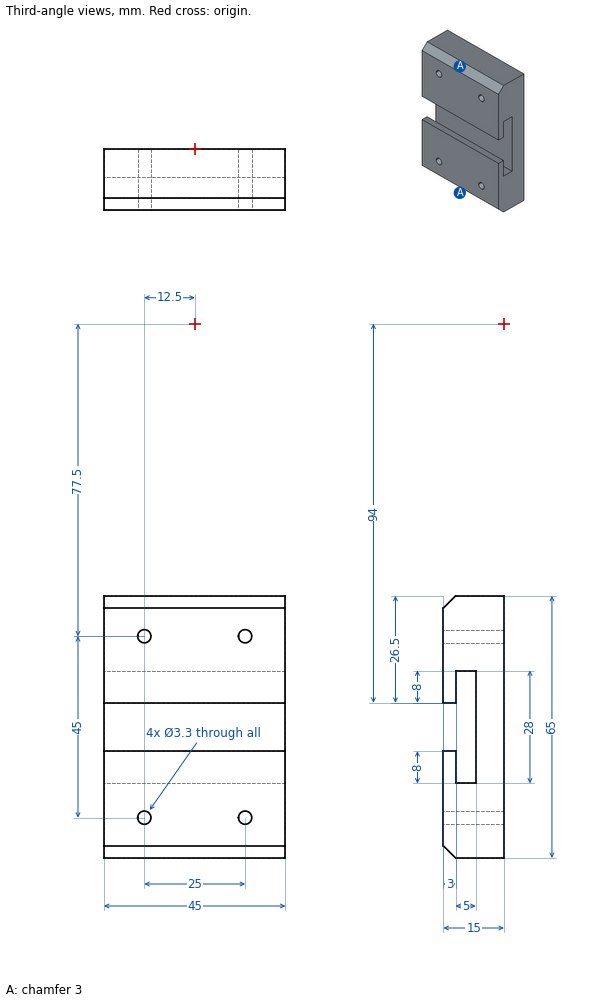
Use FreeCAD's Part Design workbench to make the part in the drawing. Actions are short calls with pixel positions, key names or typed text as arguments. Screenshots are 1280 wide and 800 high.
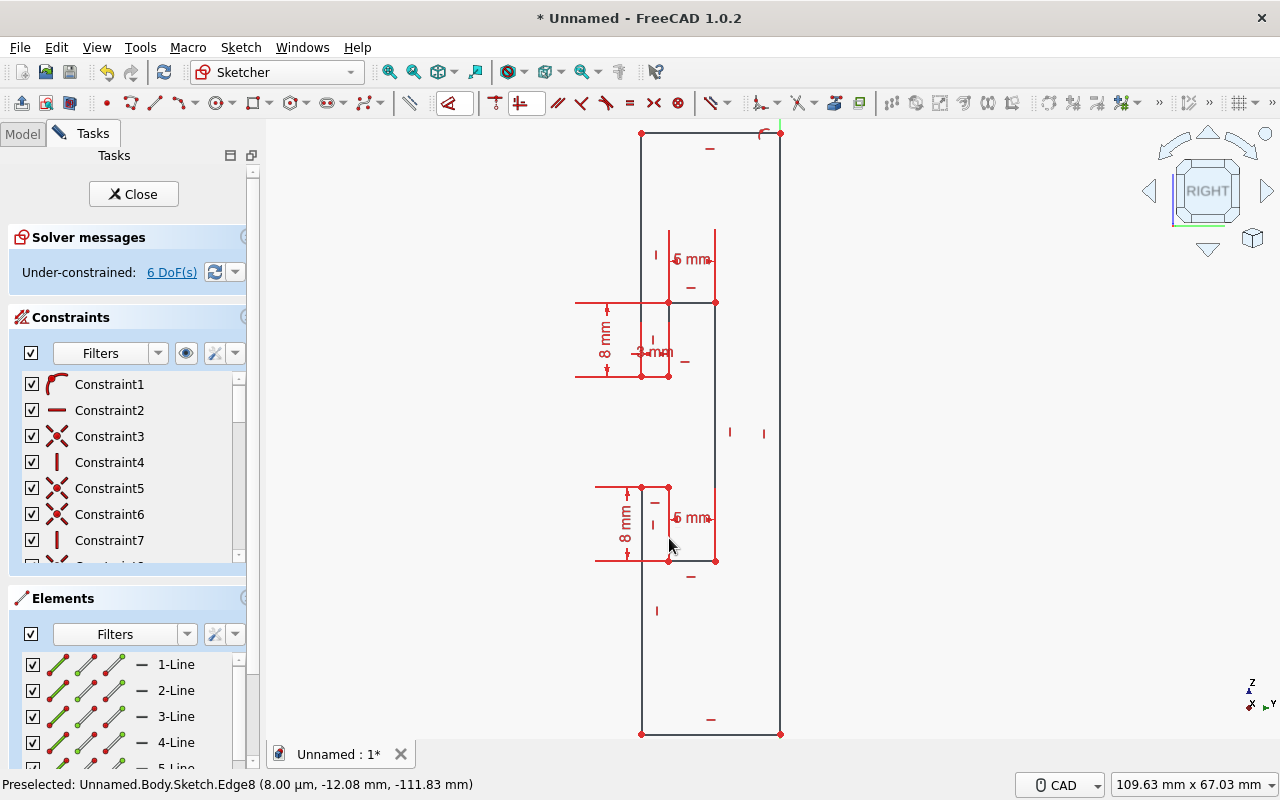
scroll(658, 487, up, 2)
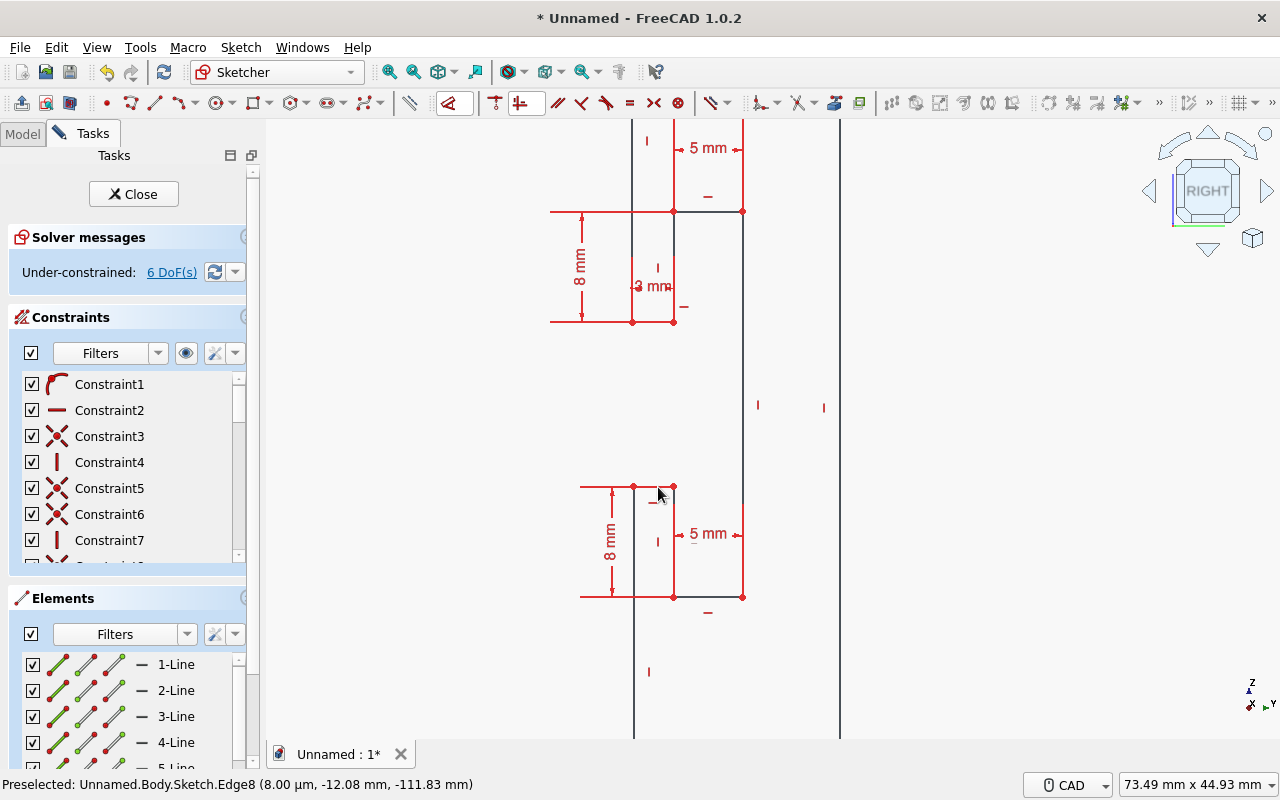
click(658, 487)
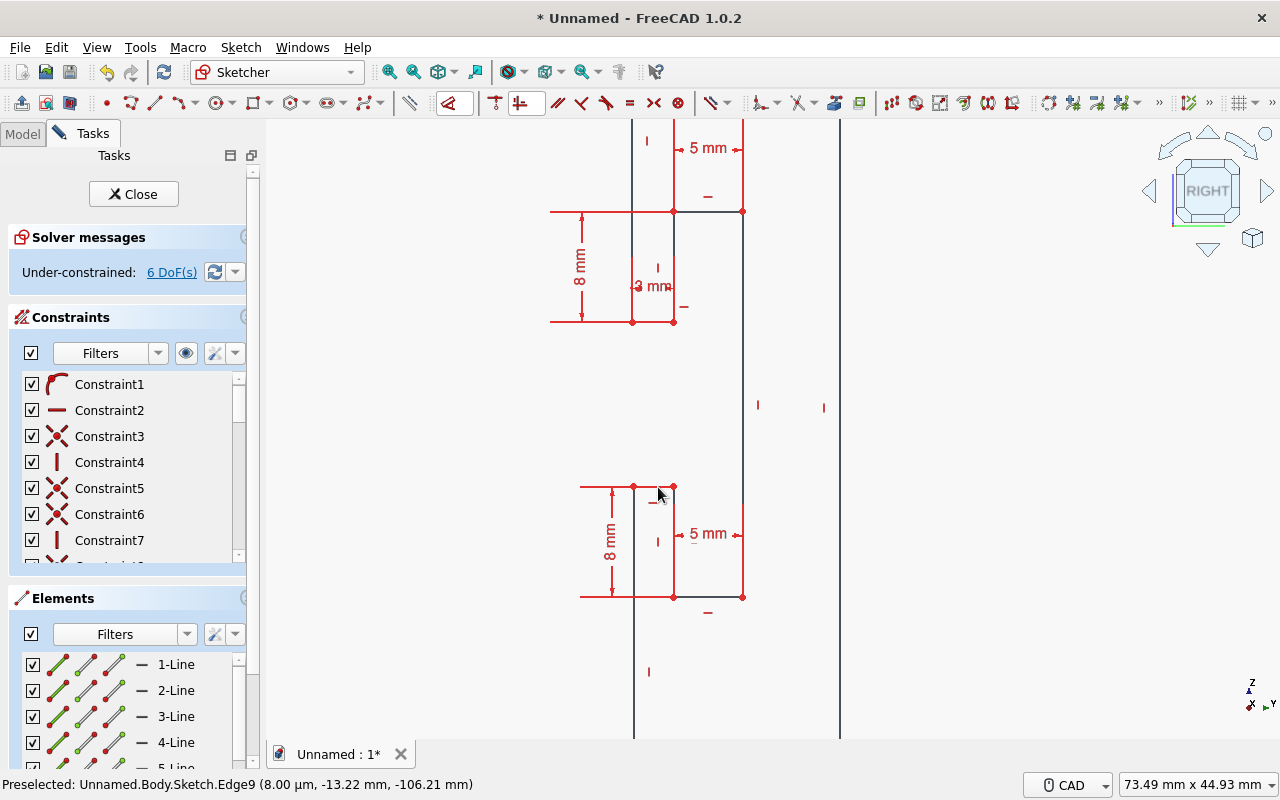
click(468, 104)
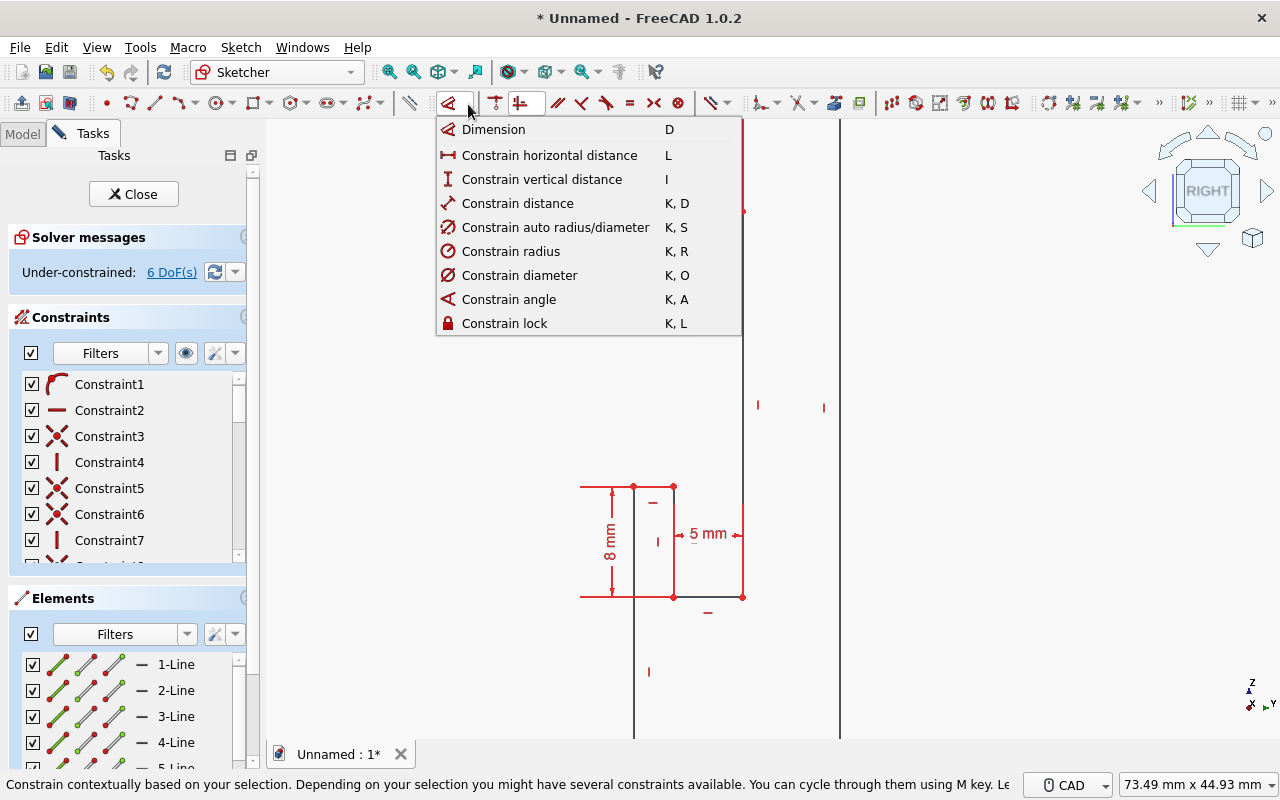
click(589, 155)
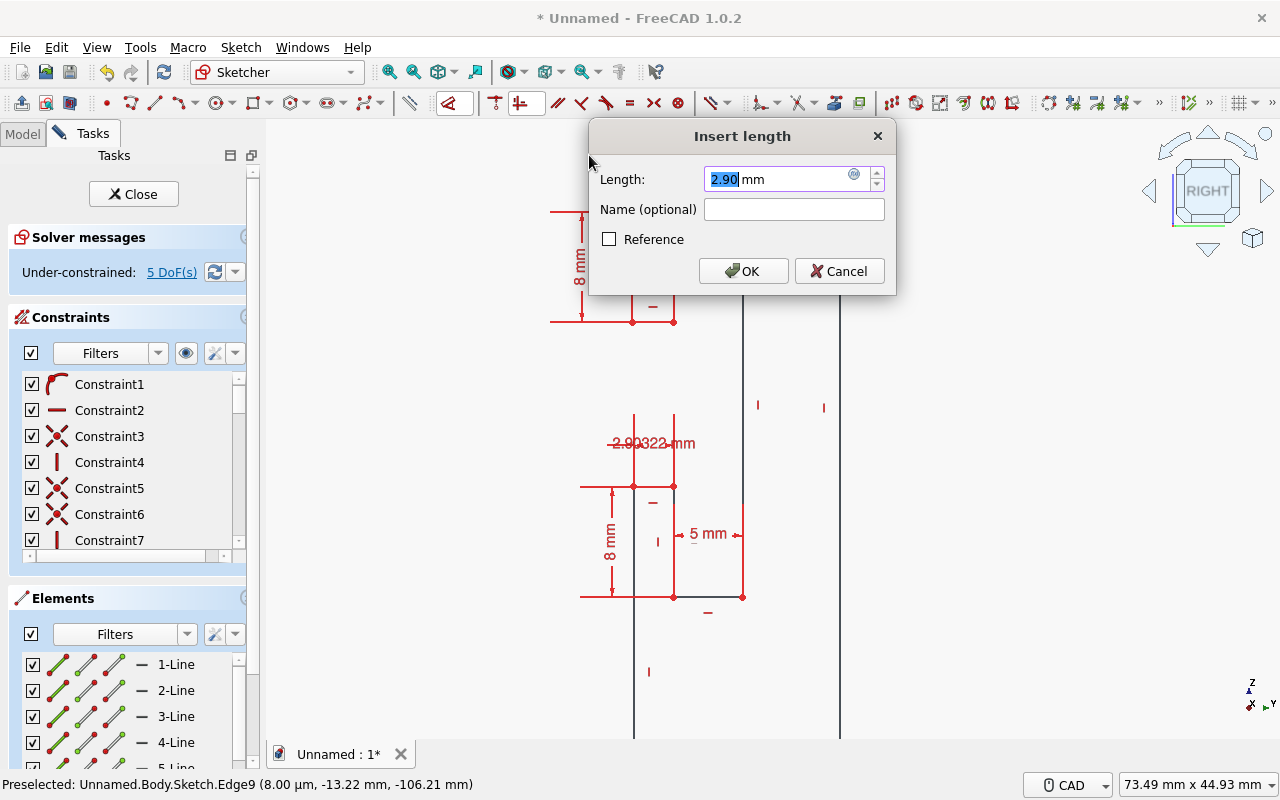
text(3)
key(Return)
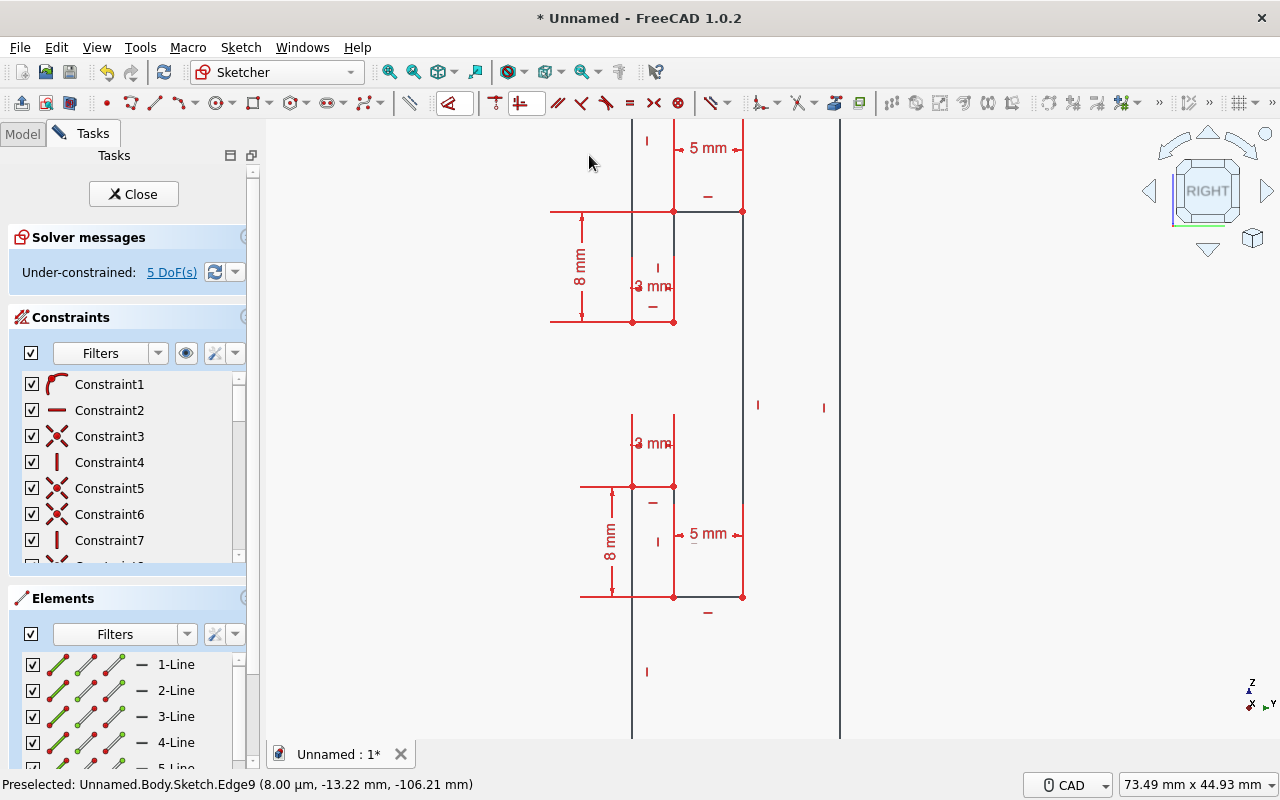
scroll(696, 554, down, 8)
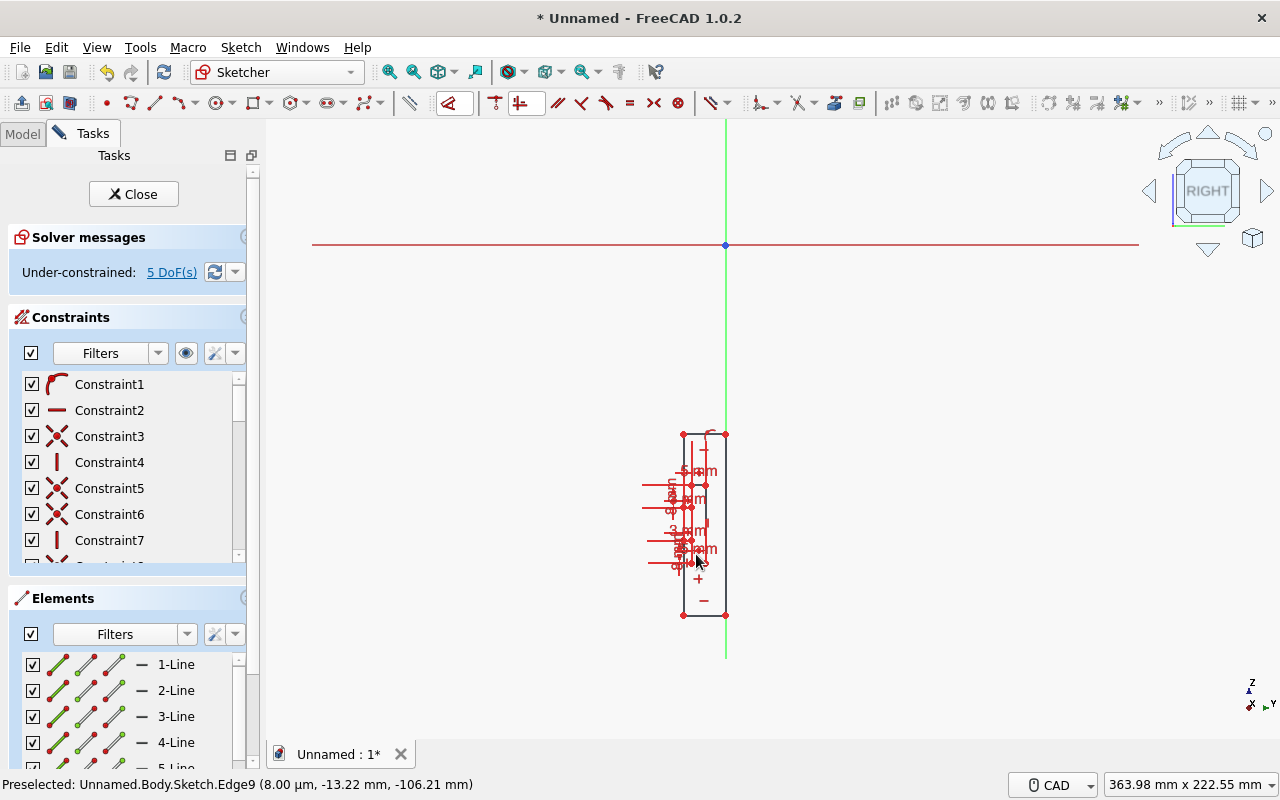
click(696, 434)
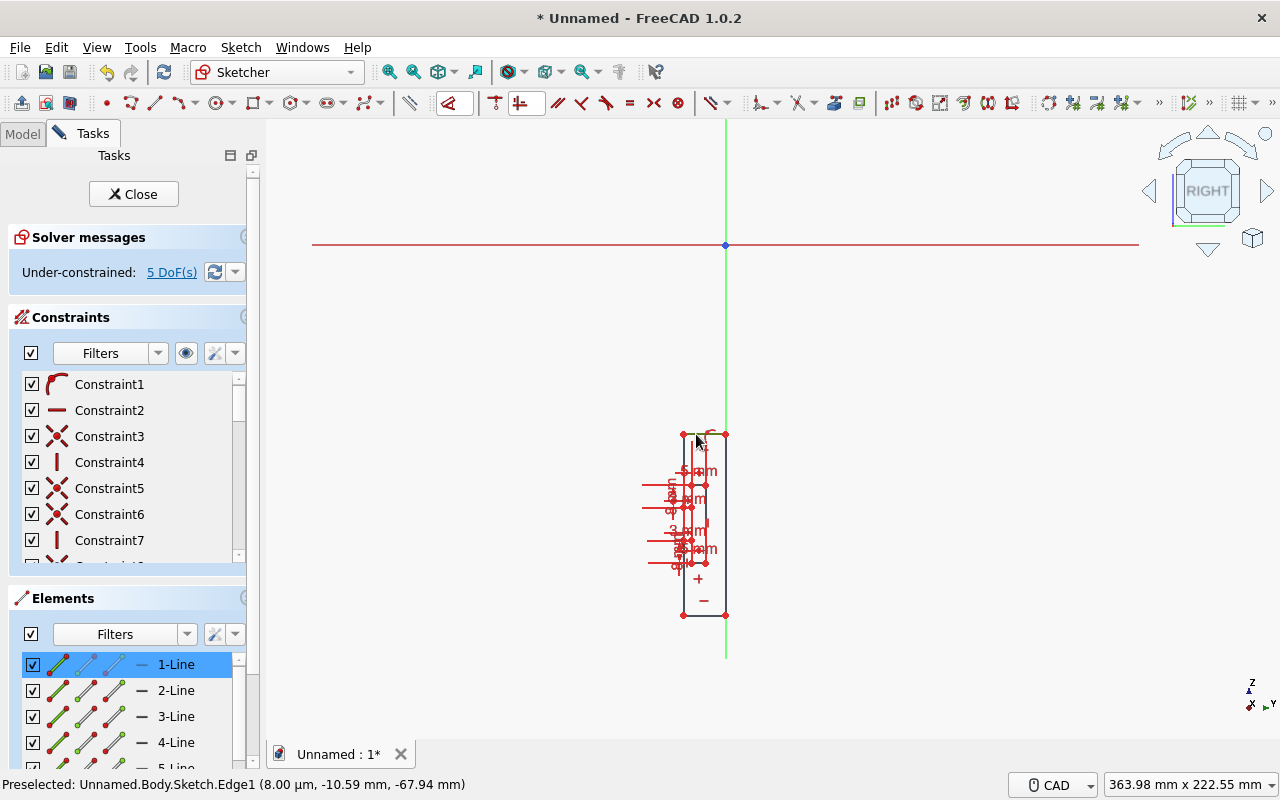
key(l)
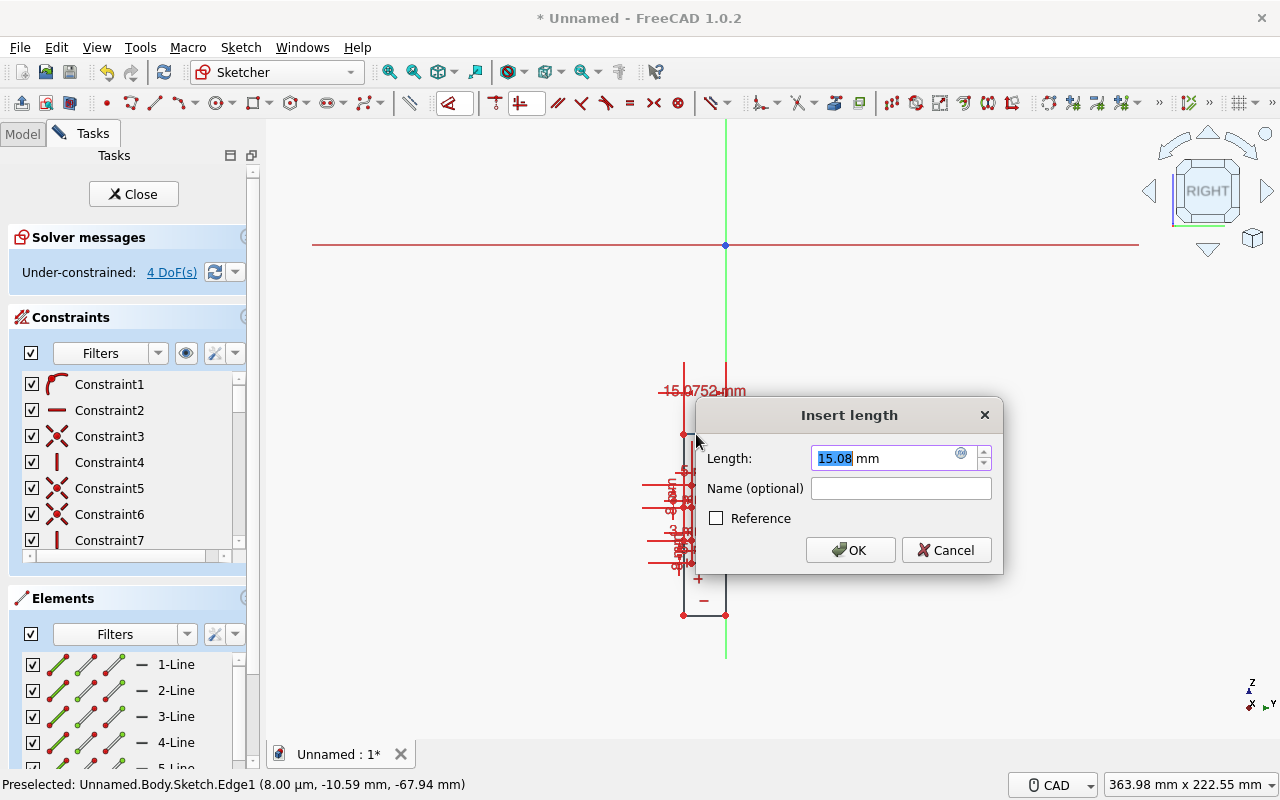
text(15)
key(Return)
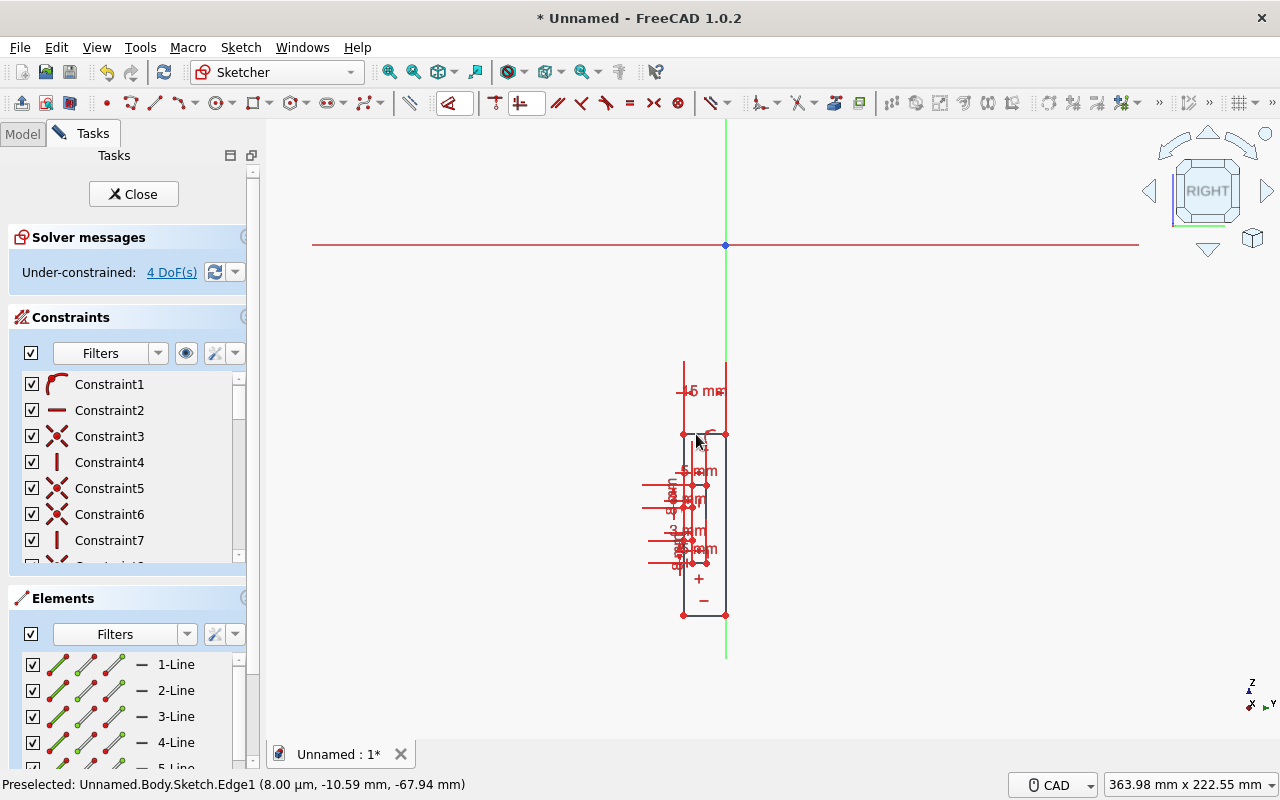
click(706, 509)